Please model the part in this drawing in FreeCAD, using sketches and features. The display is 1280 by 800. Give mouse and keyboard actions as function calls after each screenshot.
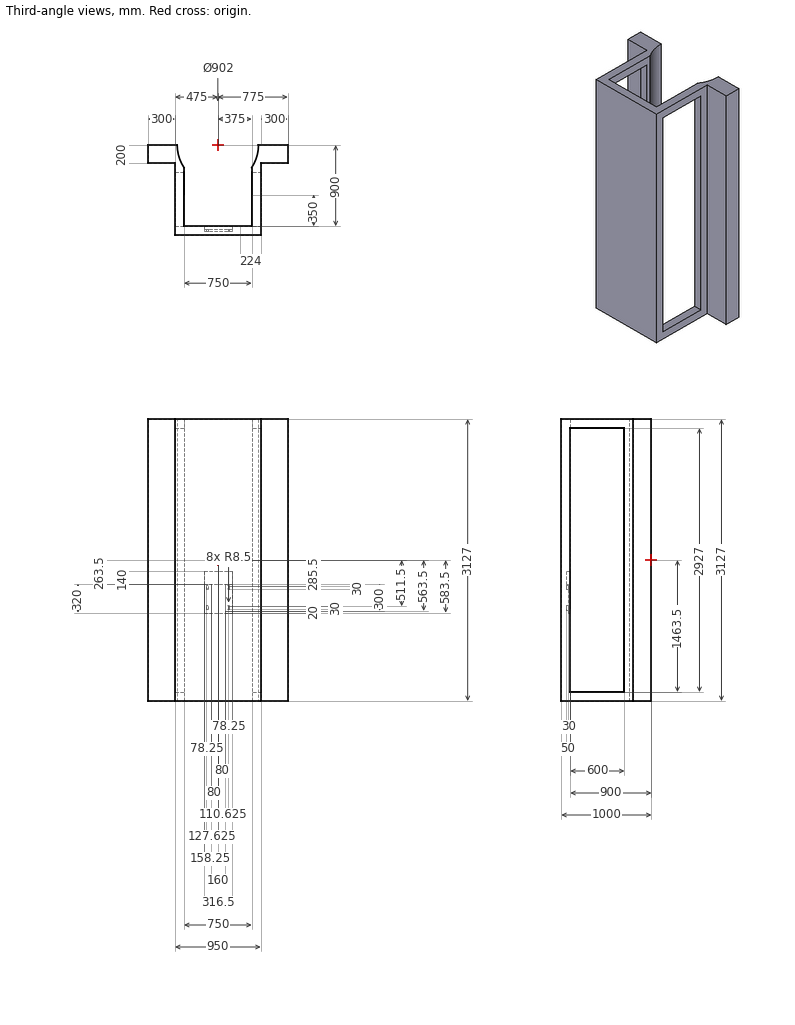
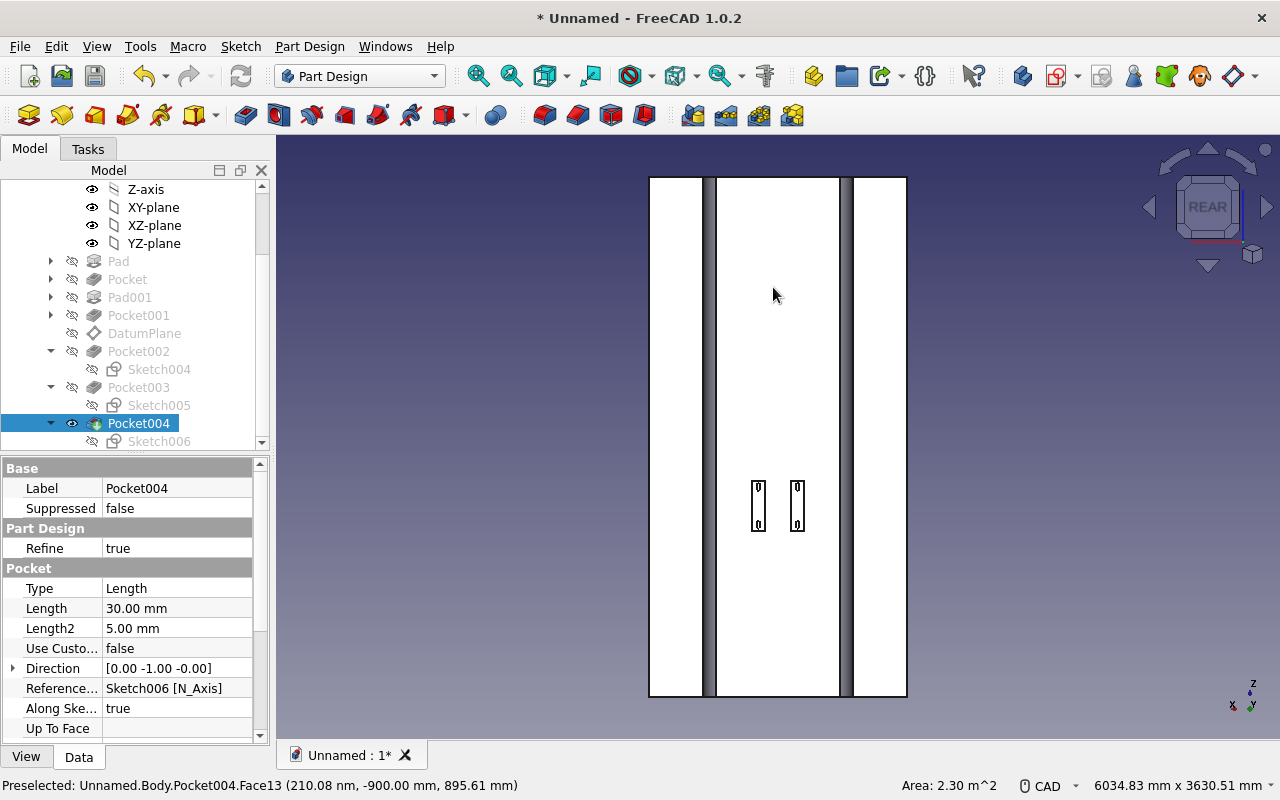
click(1056, 76)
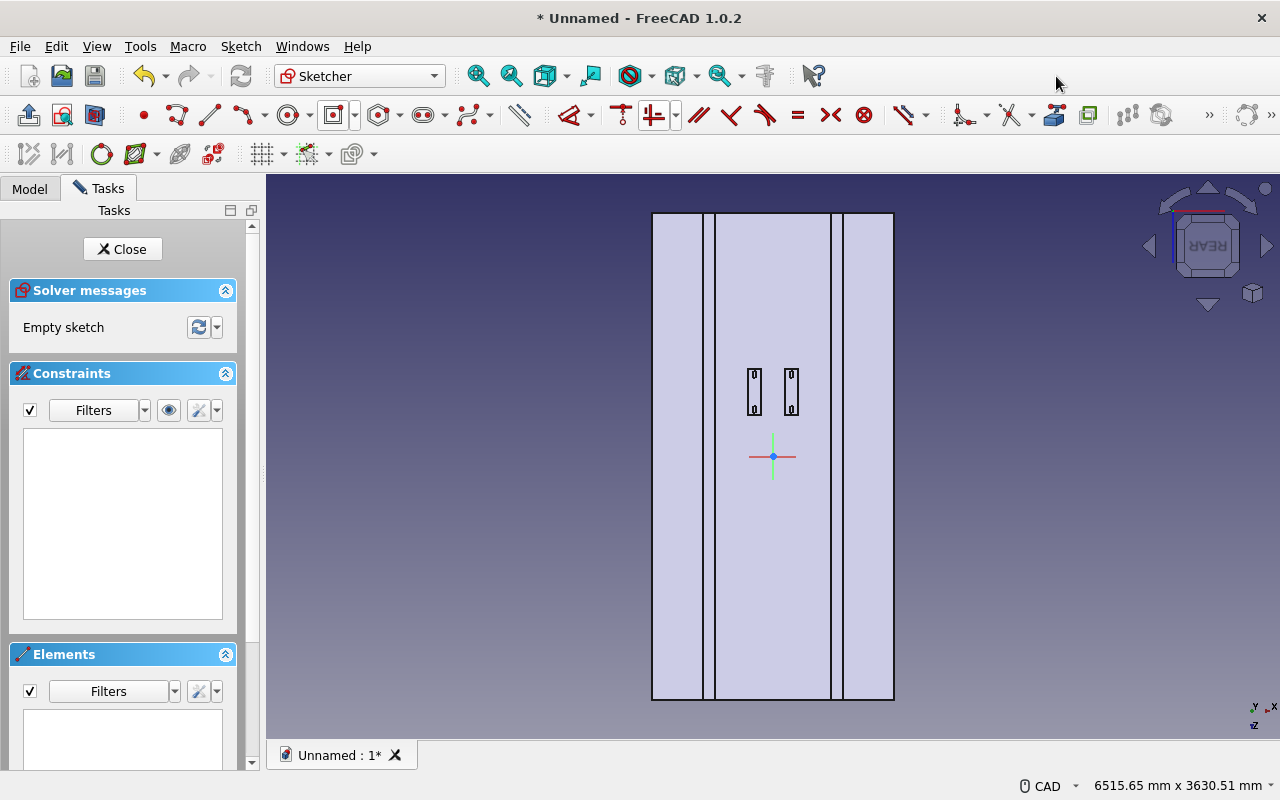
key(q)
key(s)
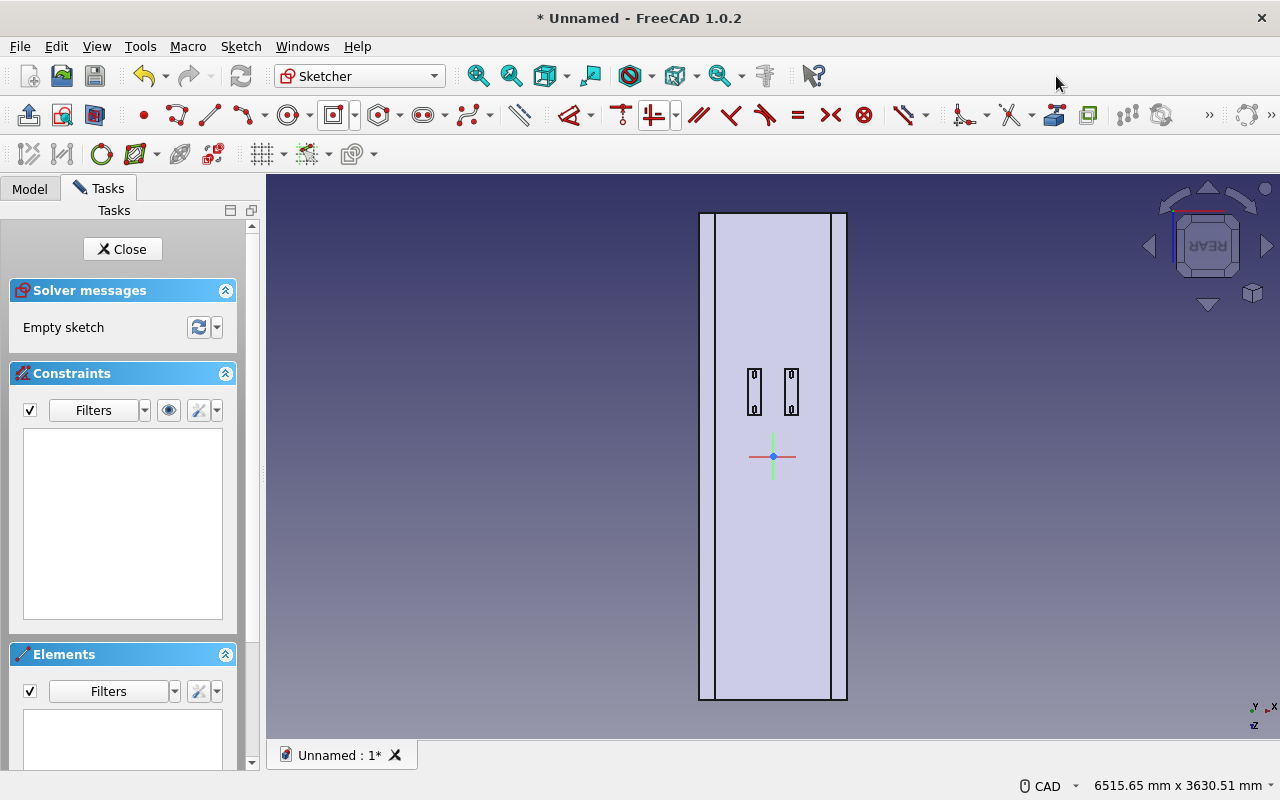
scroll(795, 396, up, 7)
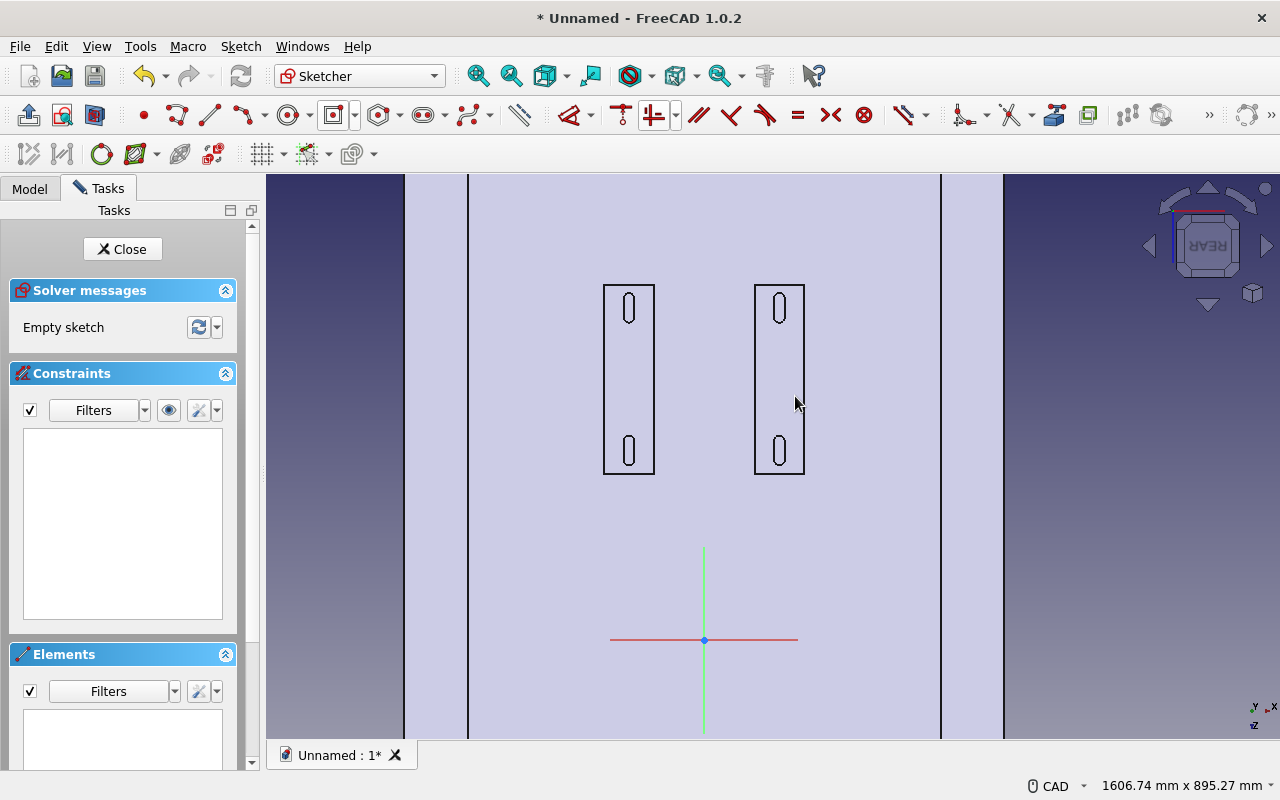
click(354, 116)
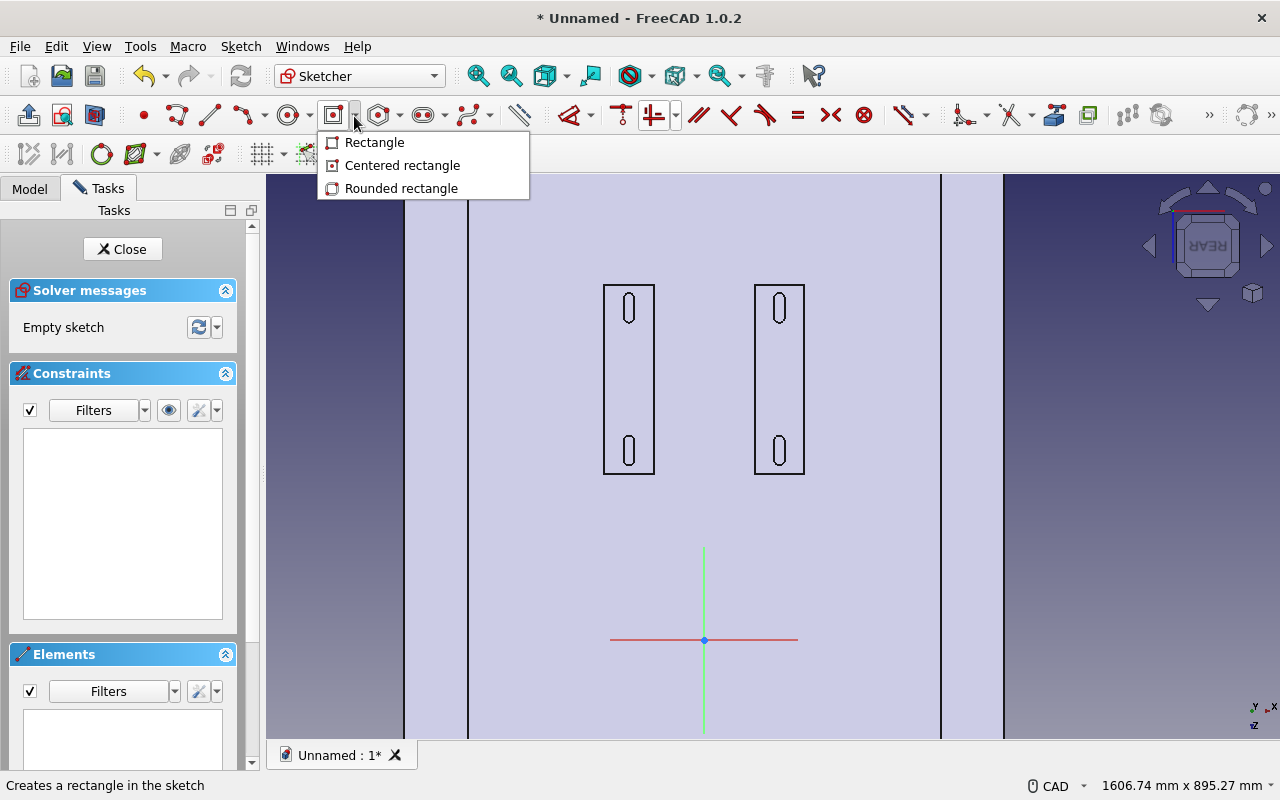
click(424, 142)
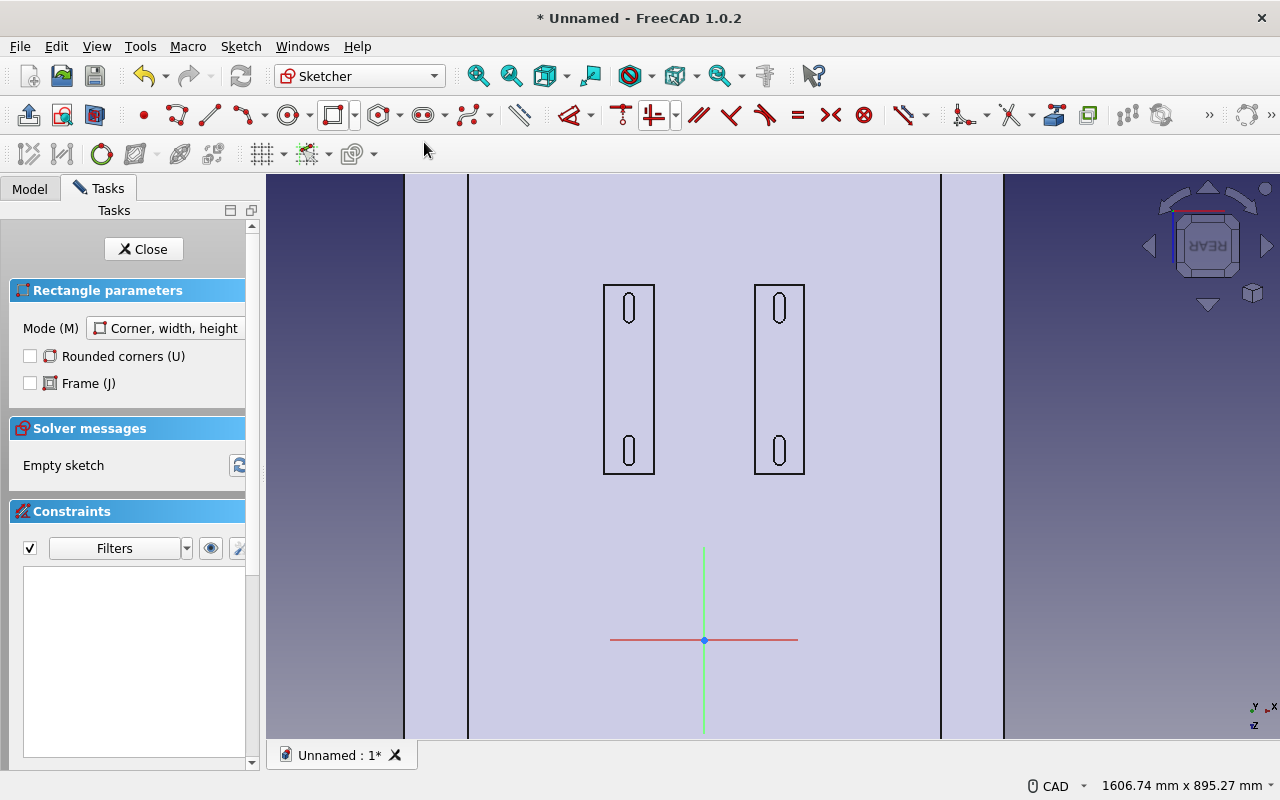
scroll(755, 272, up, 2)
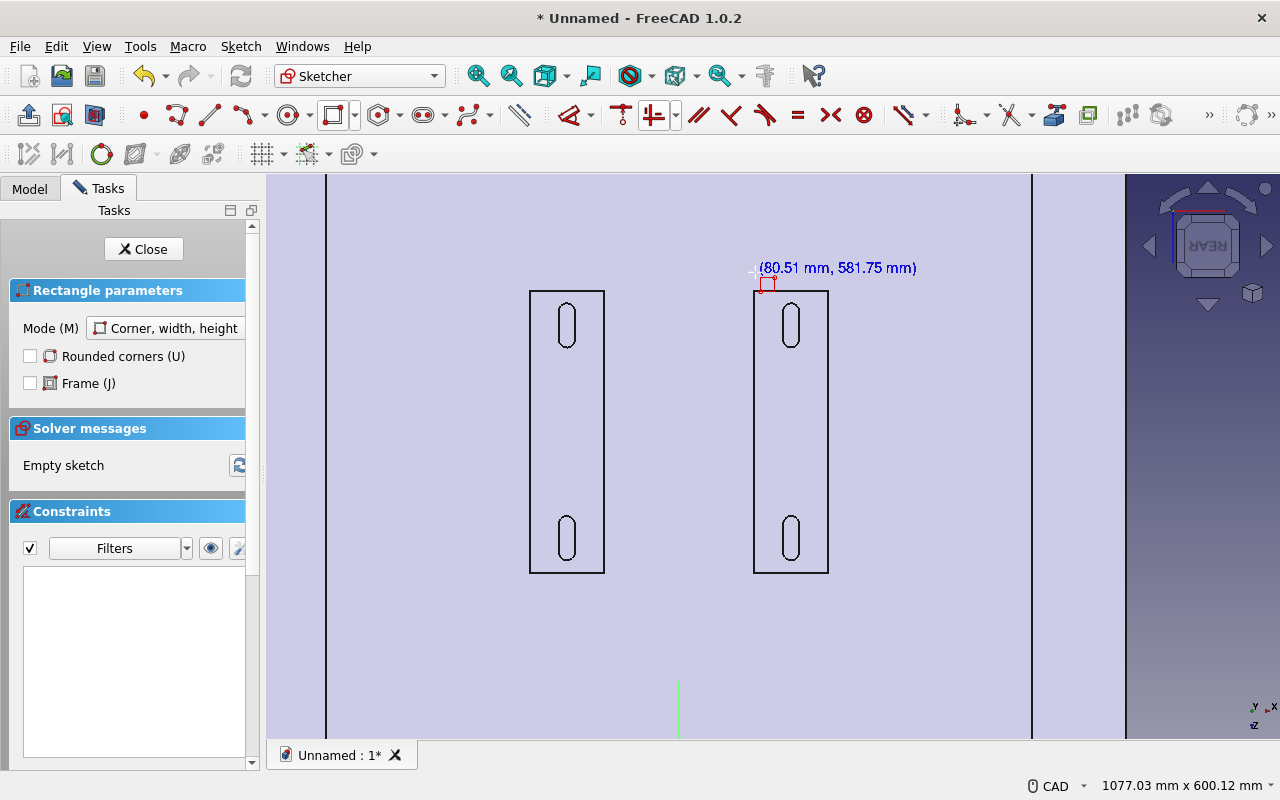
click(754, 272)
click(828, 291)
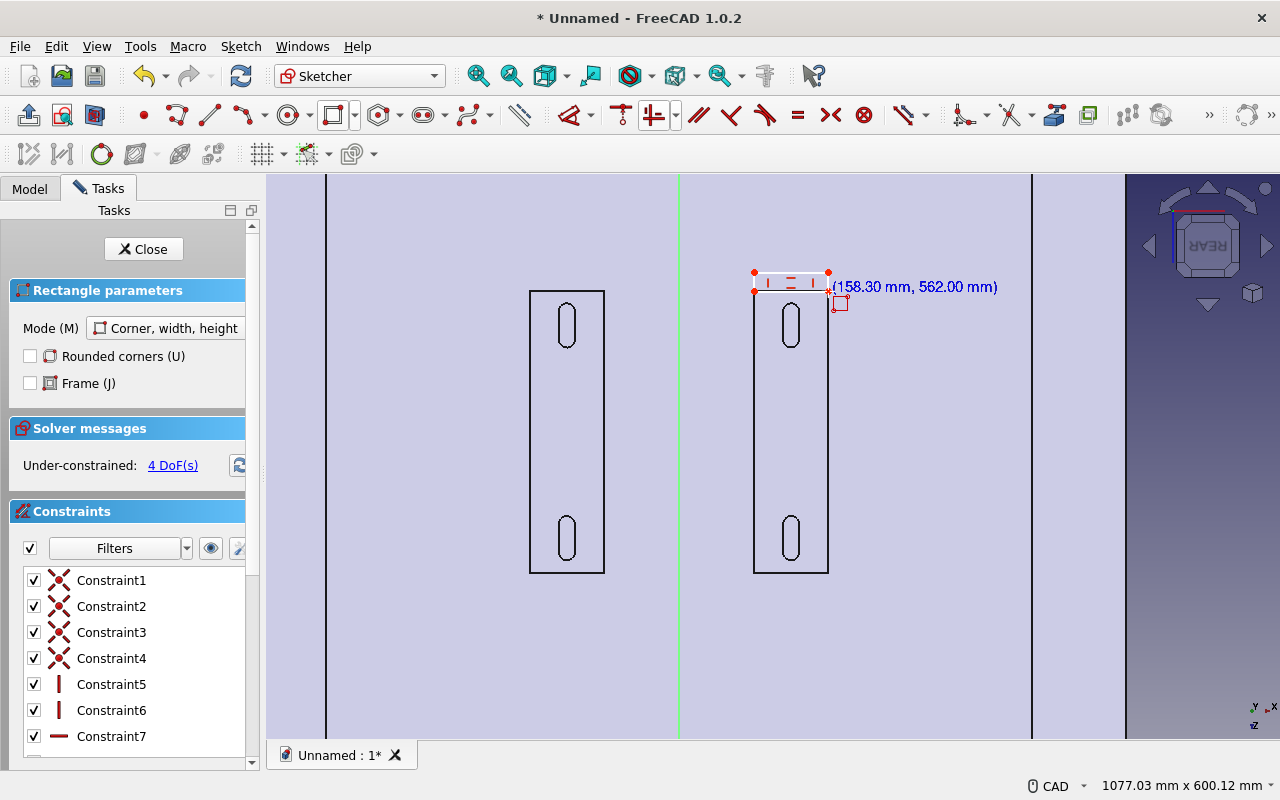
click(530, 272)
click(604, 291)
key(Escape)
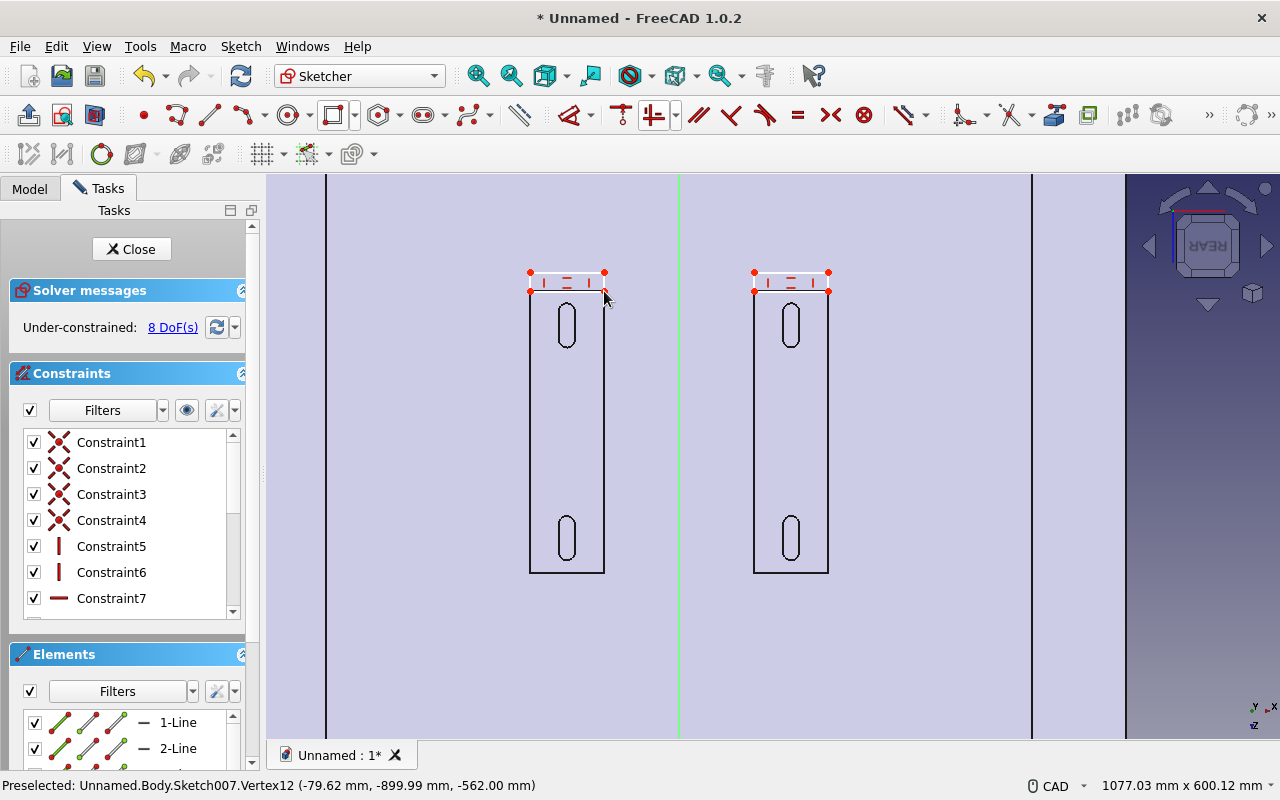
click(568, 116)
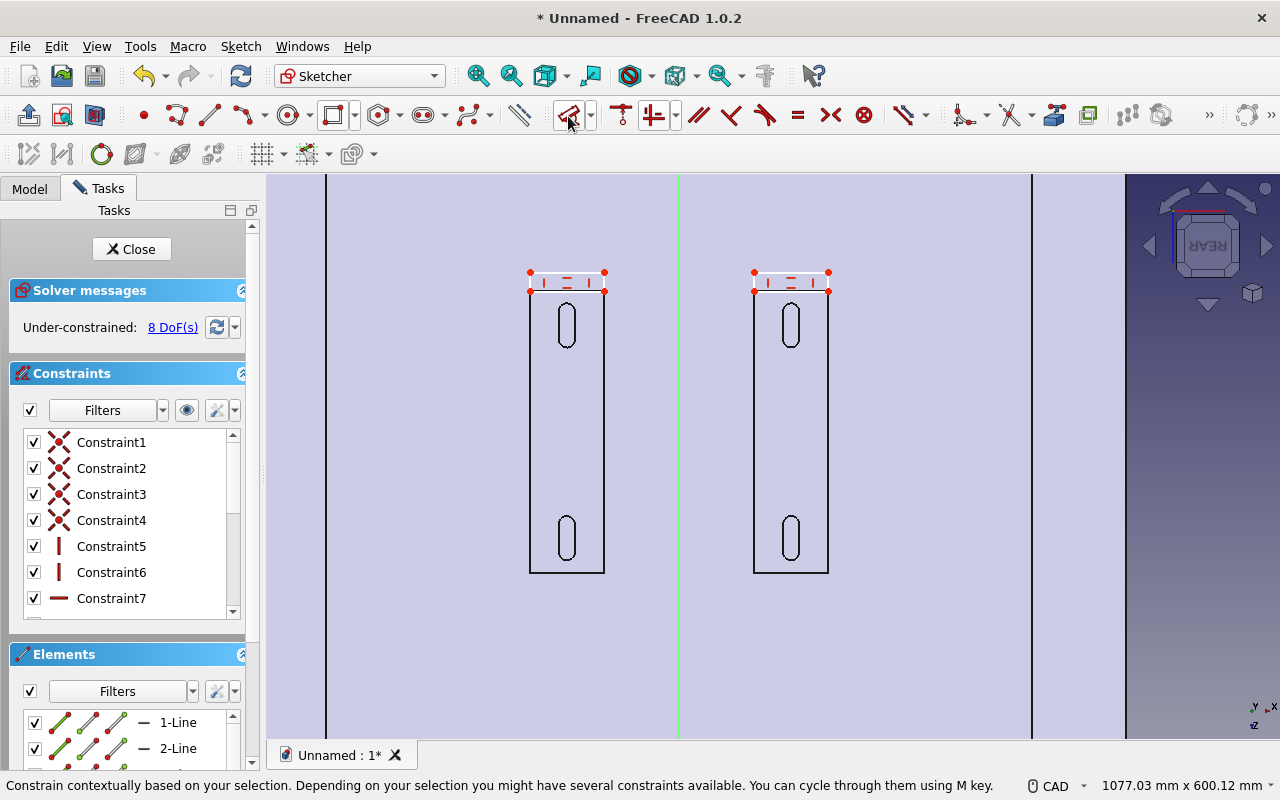
scroll(754, 283, up, 4)